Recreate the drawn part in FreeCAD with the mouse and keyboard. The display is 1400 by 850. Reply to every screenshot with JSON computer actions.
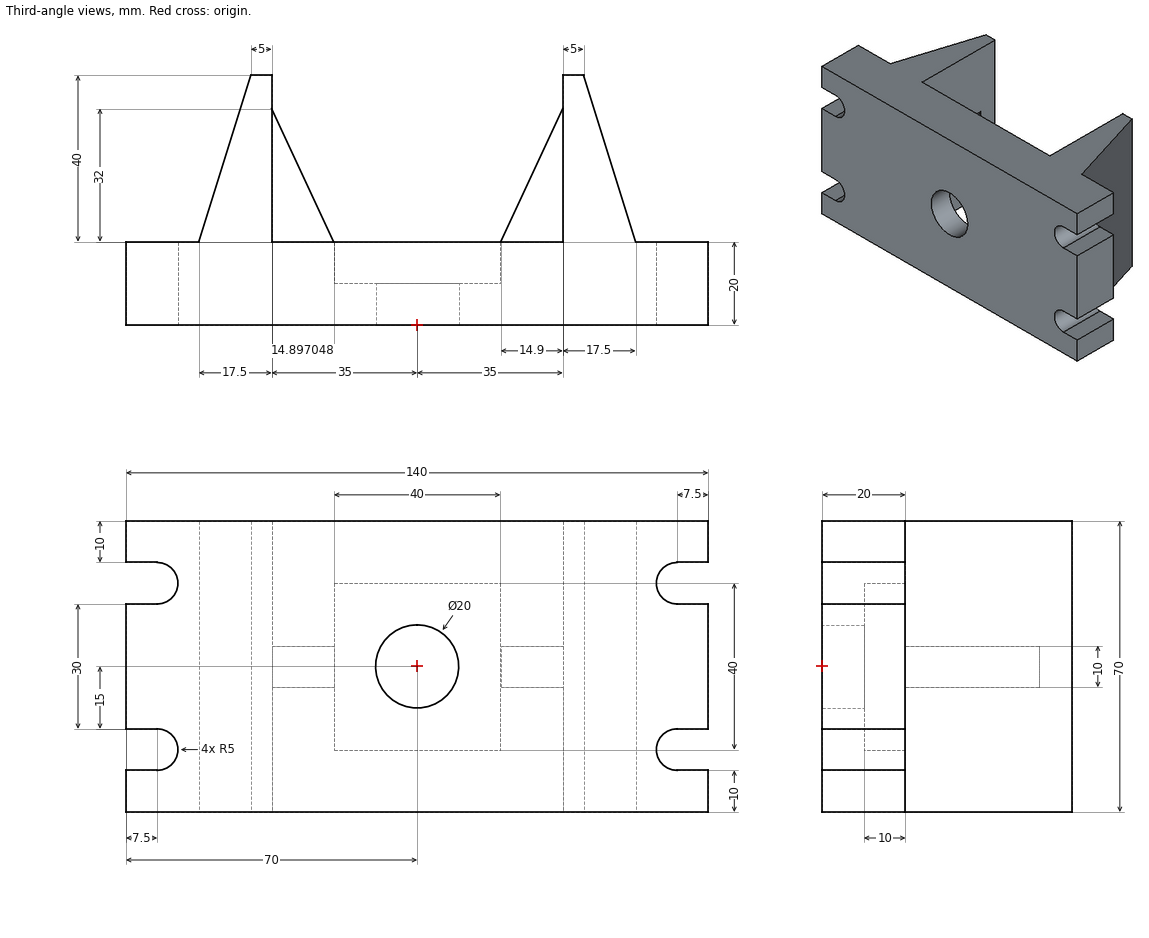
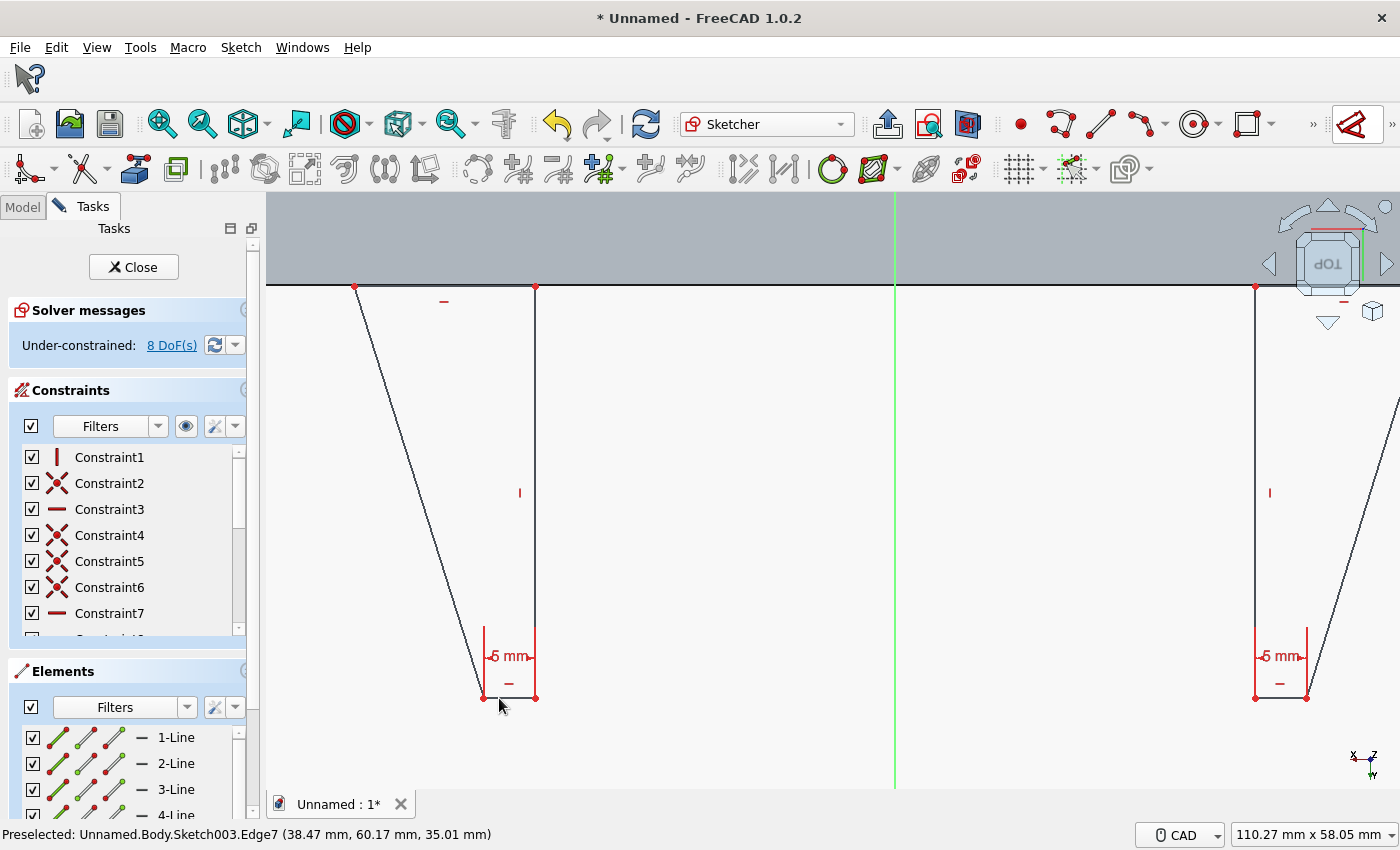
{"action": "scroll", "coordinate": [500, 699], "scroll_direction": "down", "scroll_amount": 2}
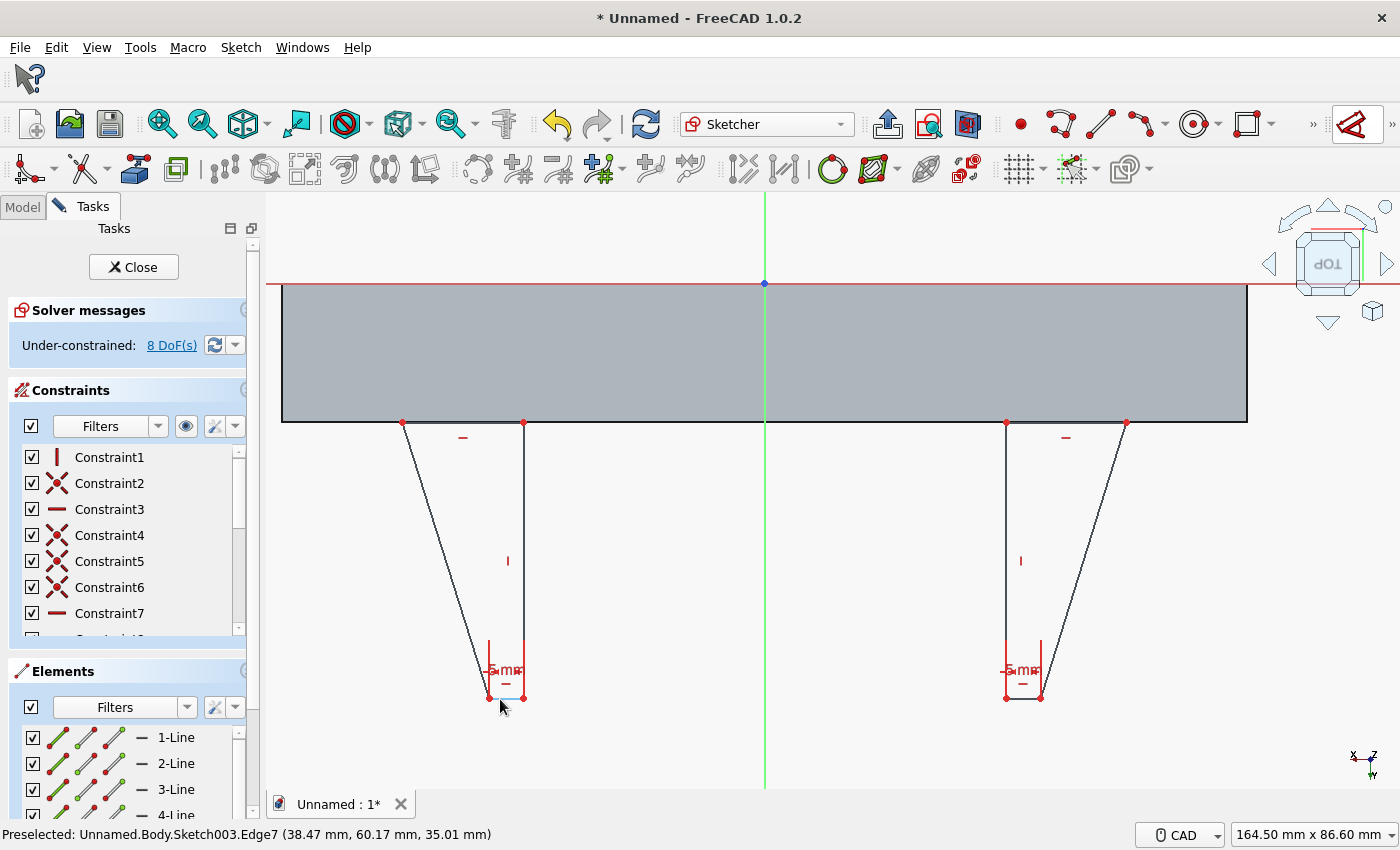
{"action": "left_click", "coordinate": [1006, 505]}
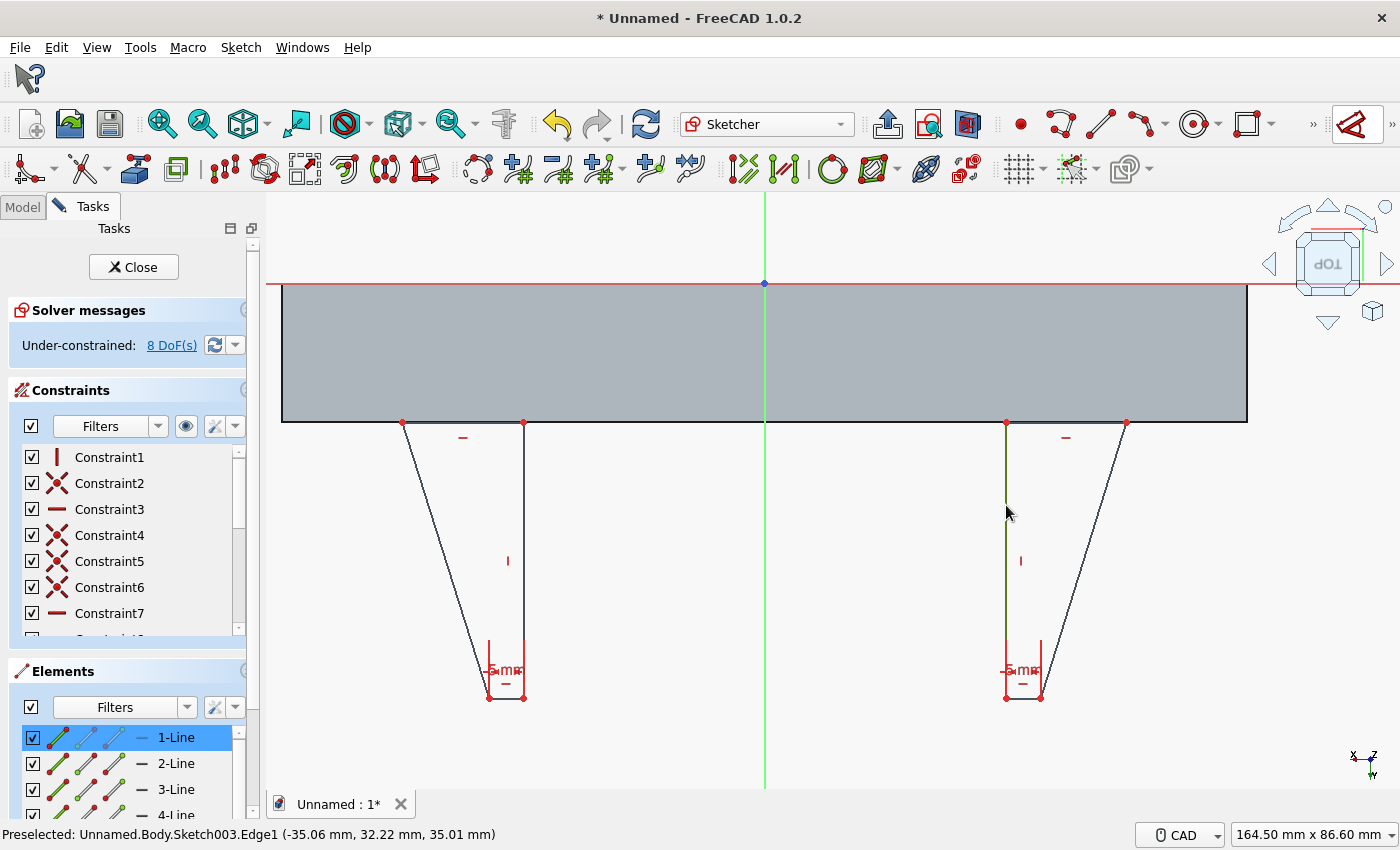
{"action": "left_click", "coordinate": [1378, 124]}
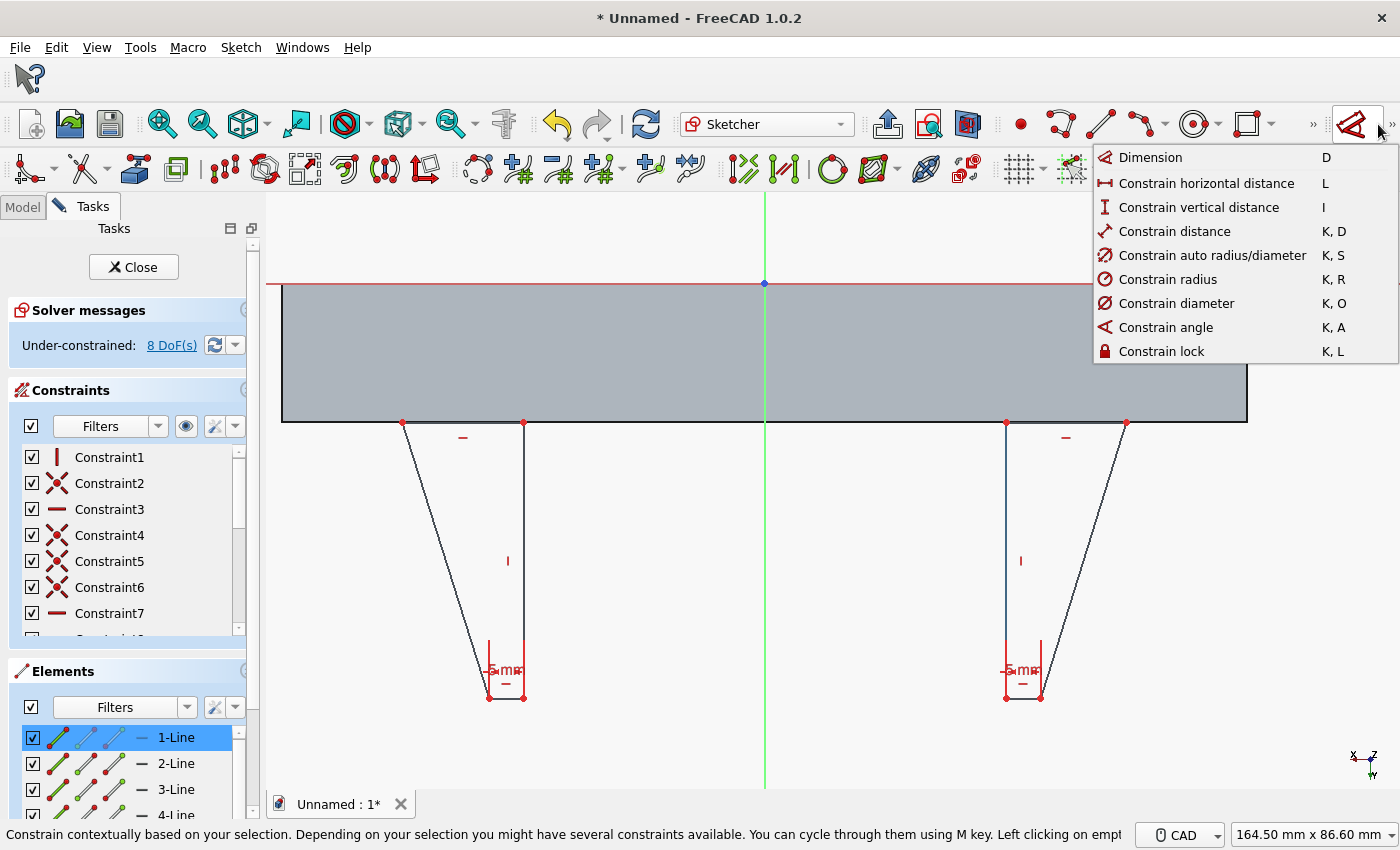
{"action": "left_click", "coordinate": [1246, 207]}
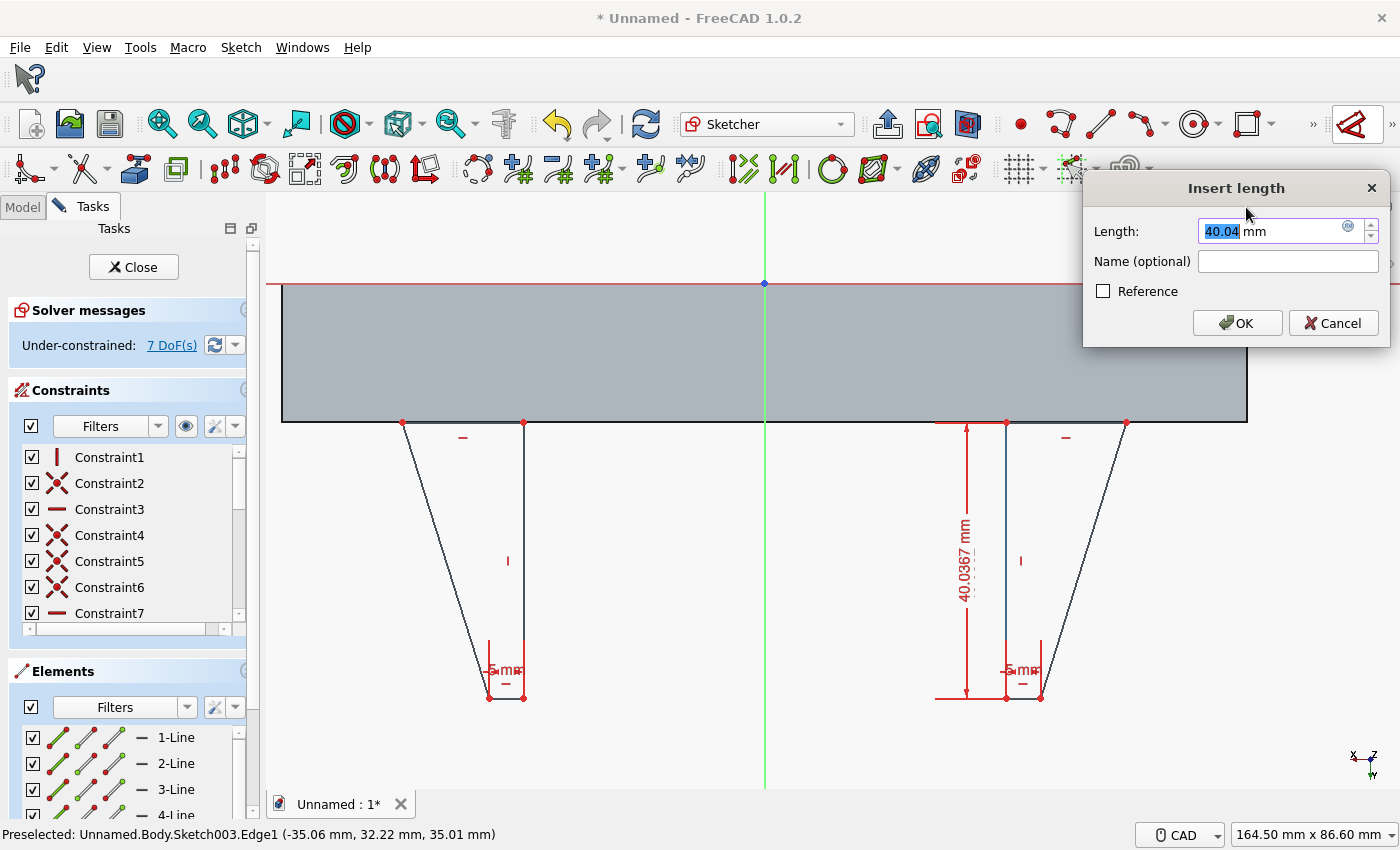
{"action": "type", "text": "40"}
{"action": "key", "text": "Return"}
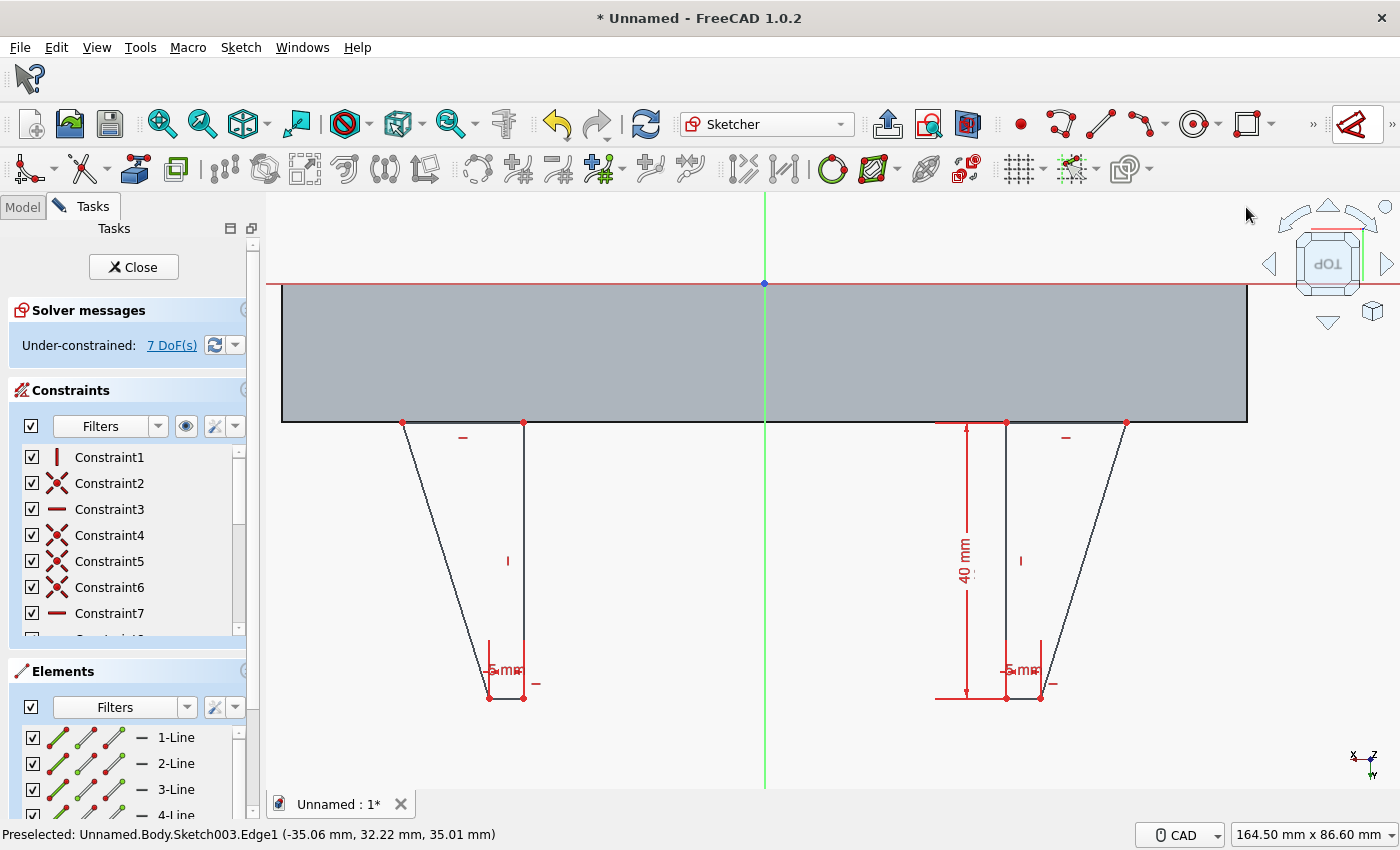
{"action": "left_click", "coordinate": [524, 616]}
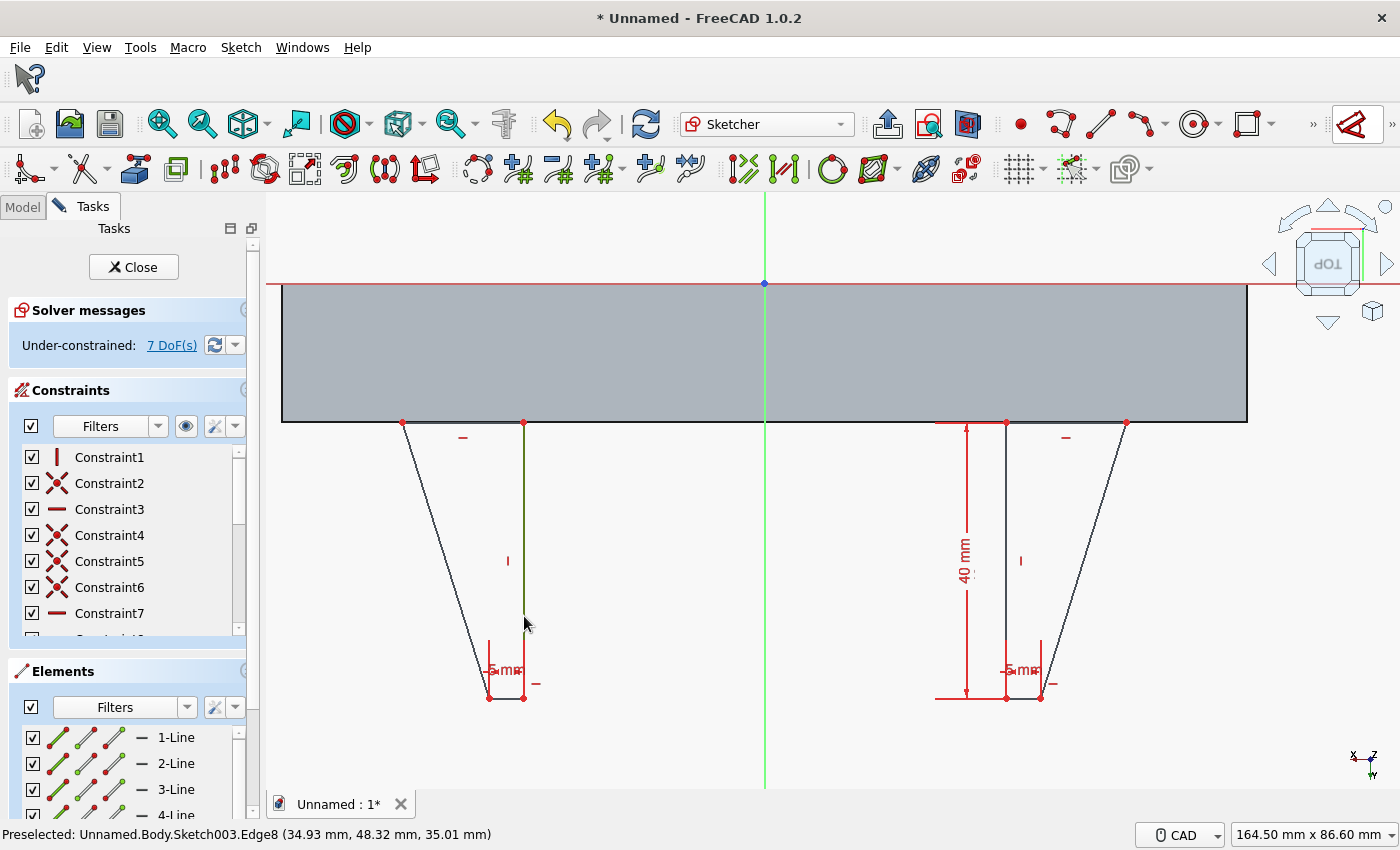
{"action": "left_click", "coordinate": [1378, 124]}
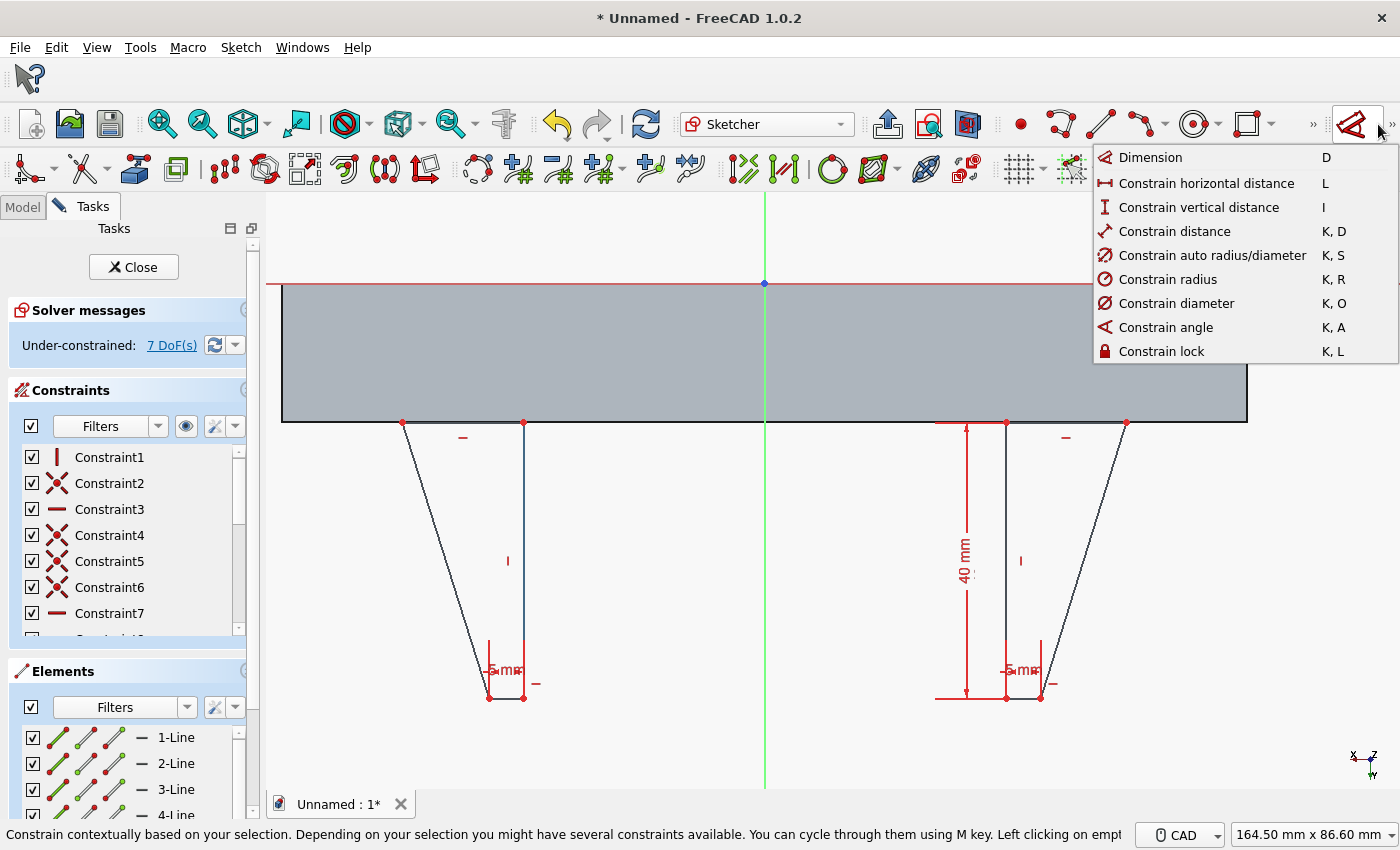
{"action": "left_click", "coordinate": [1246, 207]}